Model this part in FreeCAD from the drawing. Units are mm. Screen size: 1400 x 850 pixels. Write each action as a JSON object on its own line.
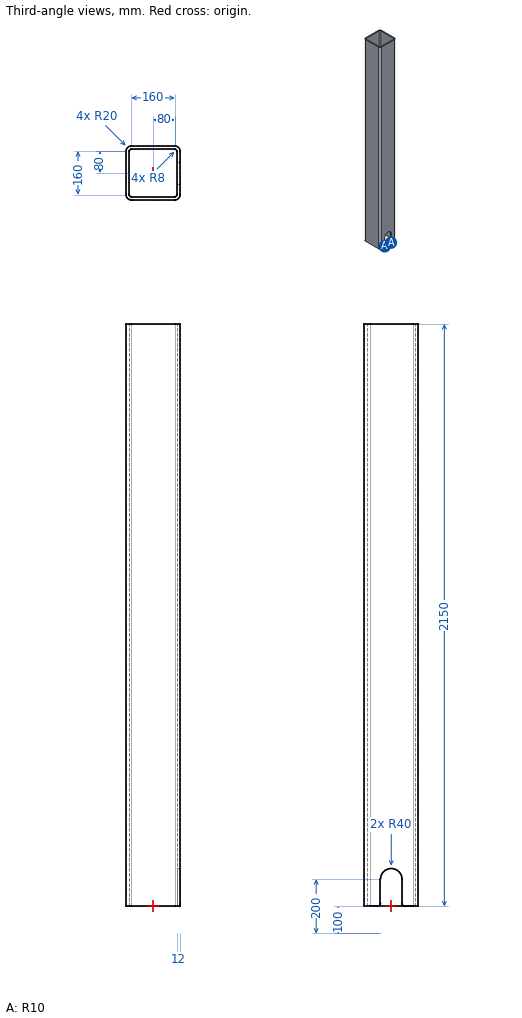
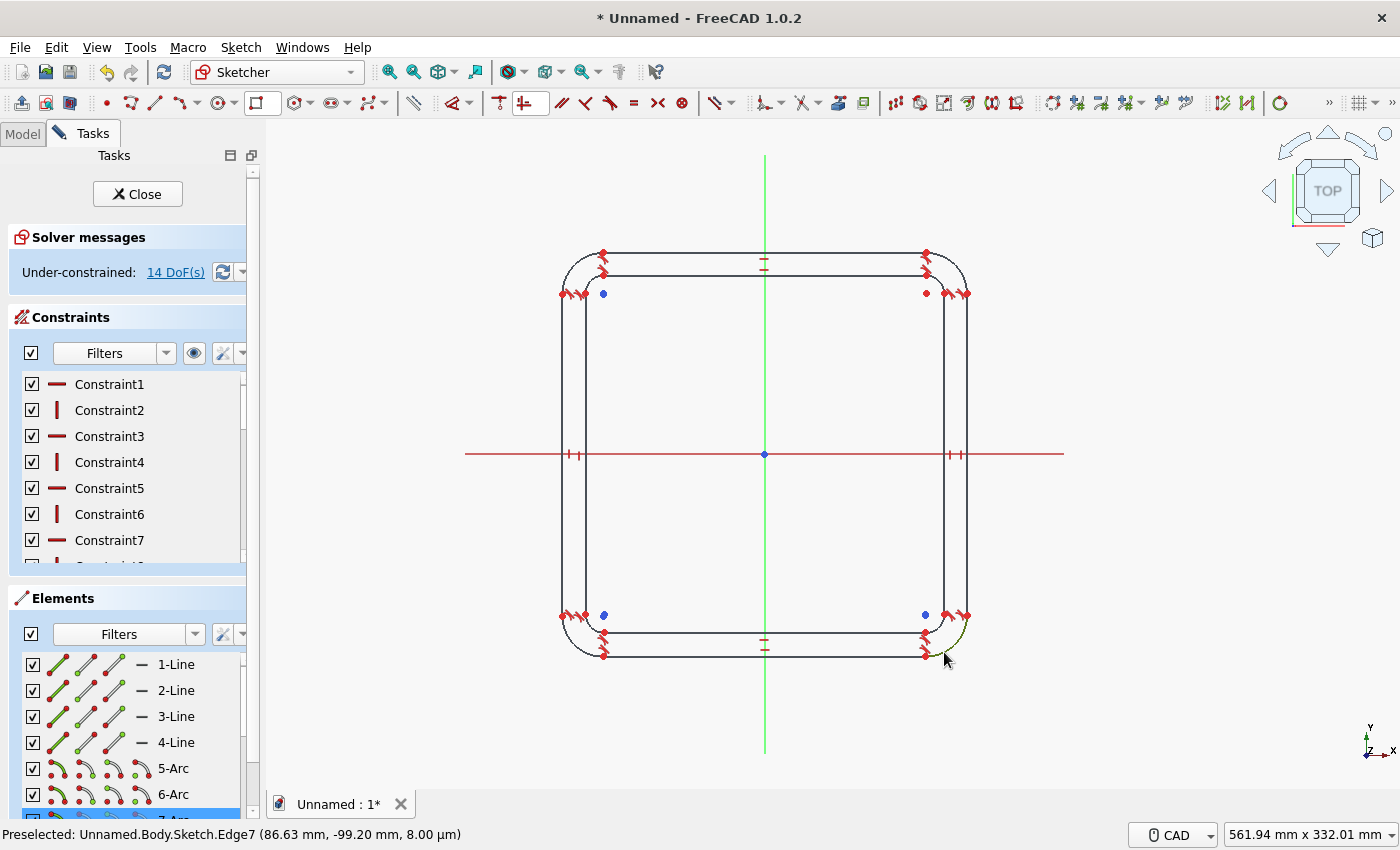
{"action": "left_click", "coordinate": [939, 628]}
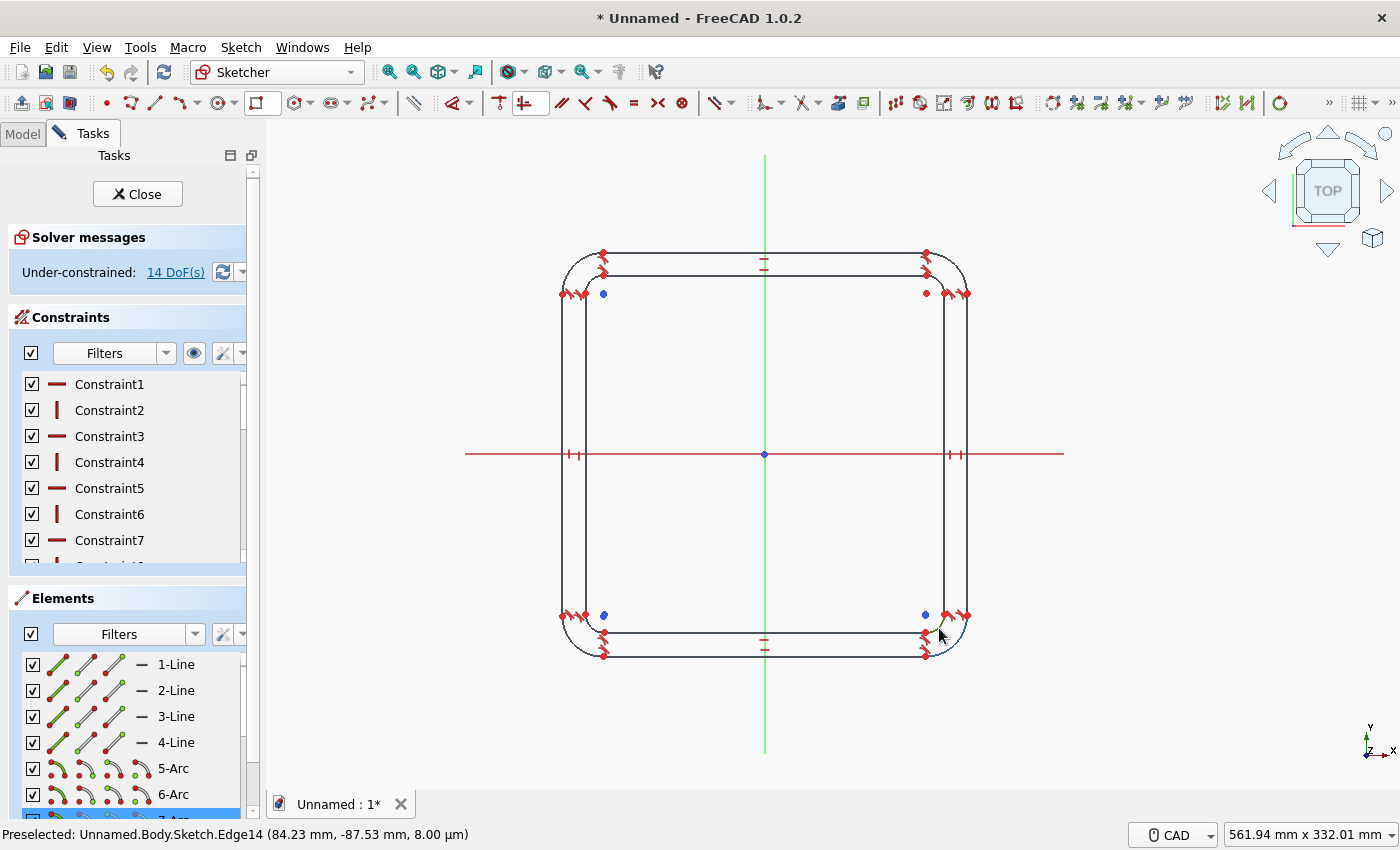
{"action": "left_click", "coordinate": [500, 104]}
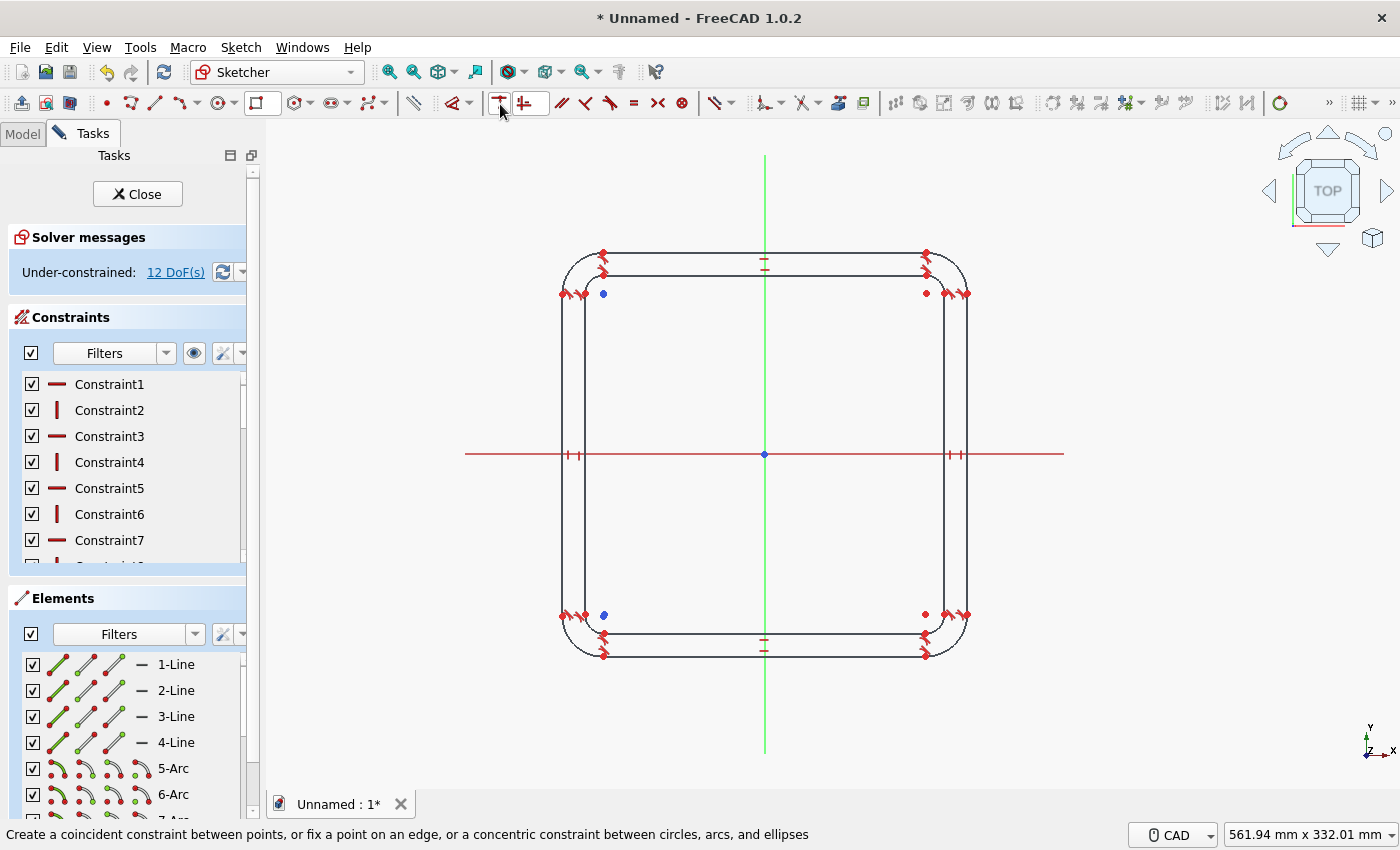
{"action": "left_click", "coordinate": [567, 635]}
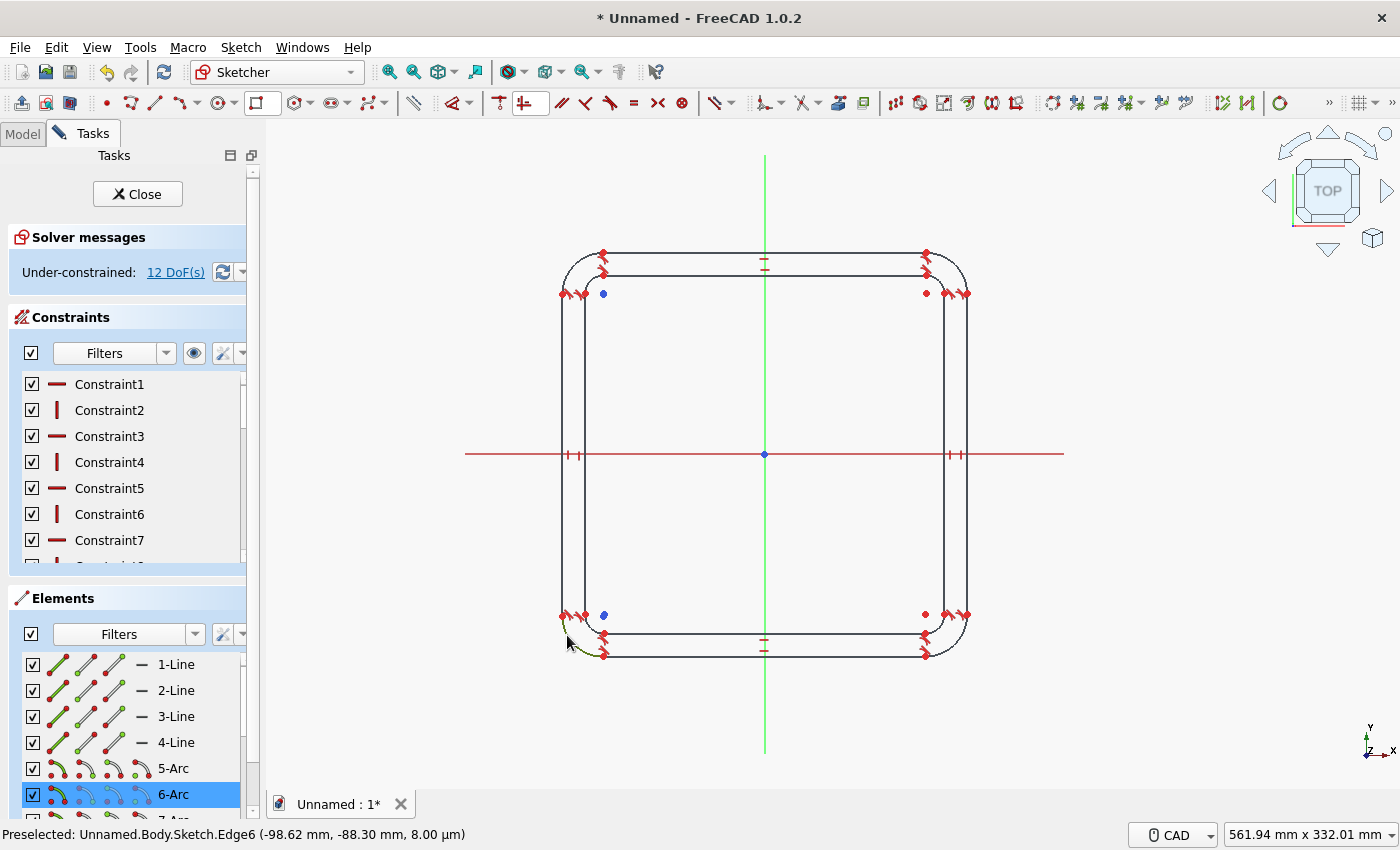
{"action": "scroll", "coordinate": [587, 623], "scroll_direction": "up", "scroll_amount": 3}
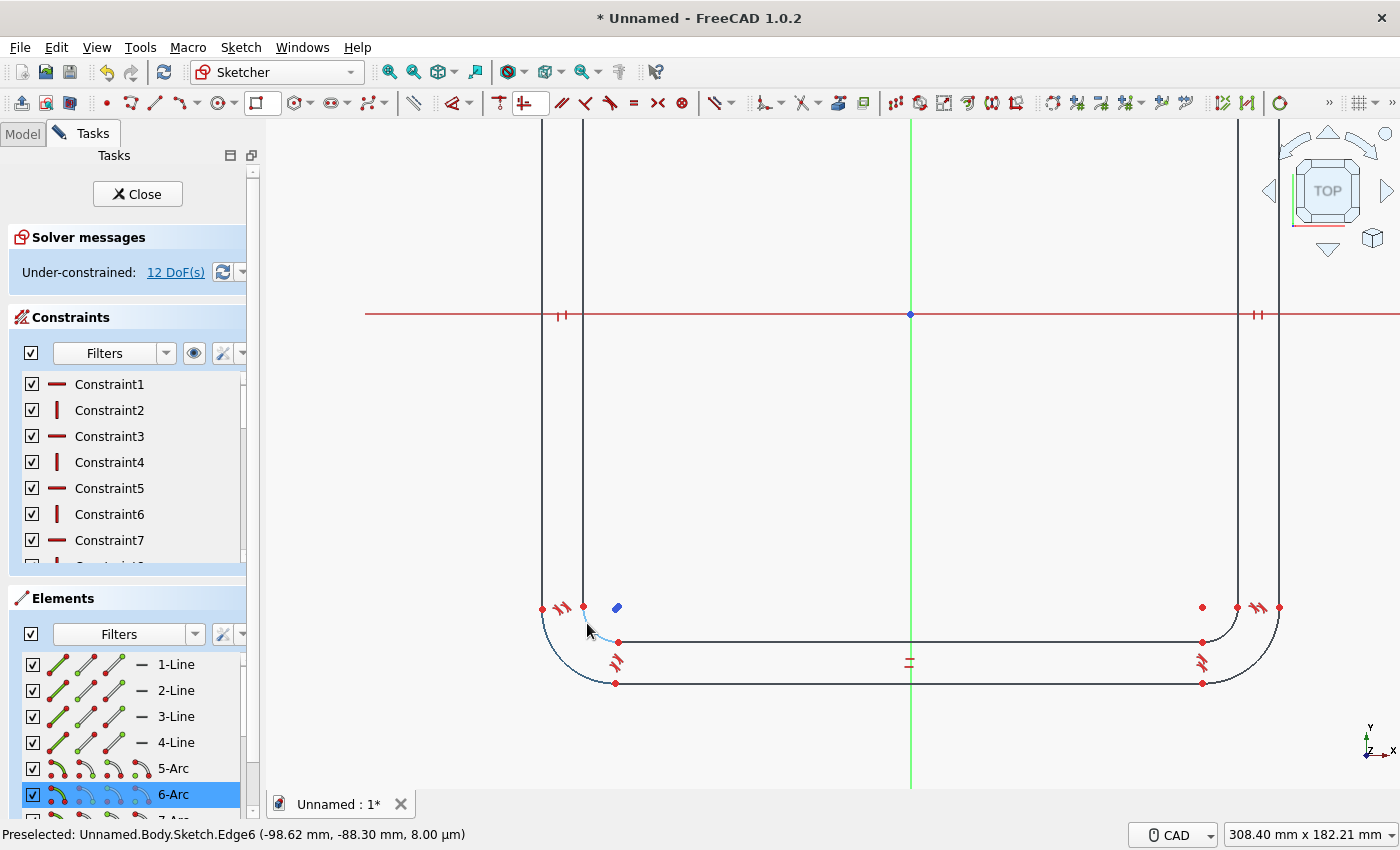
{"action": "left_click", "coordinate": [587, 623]}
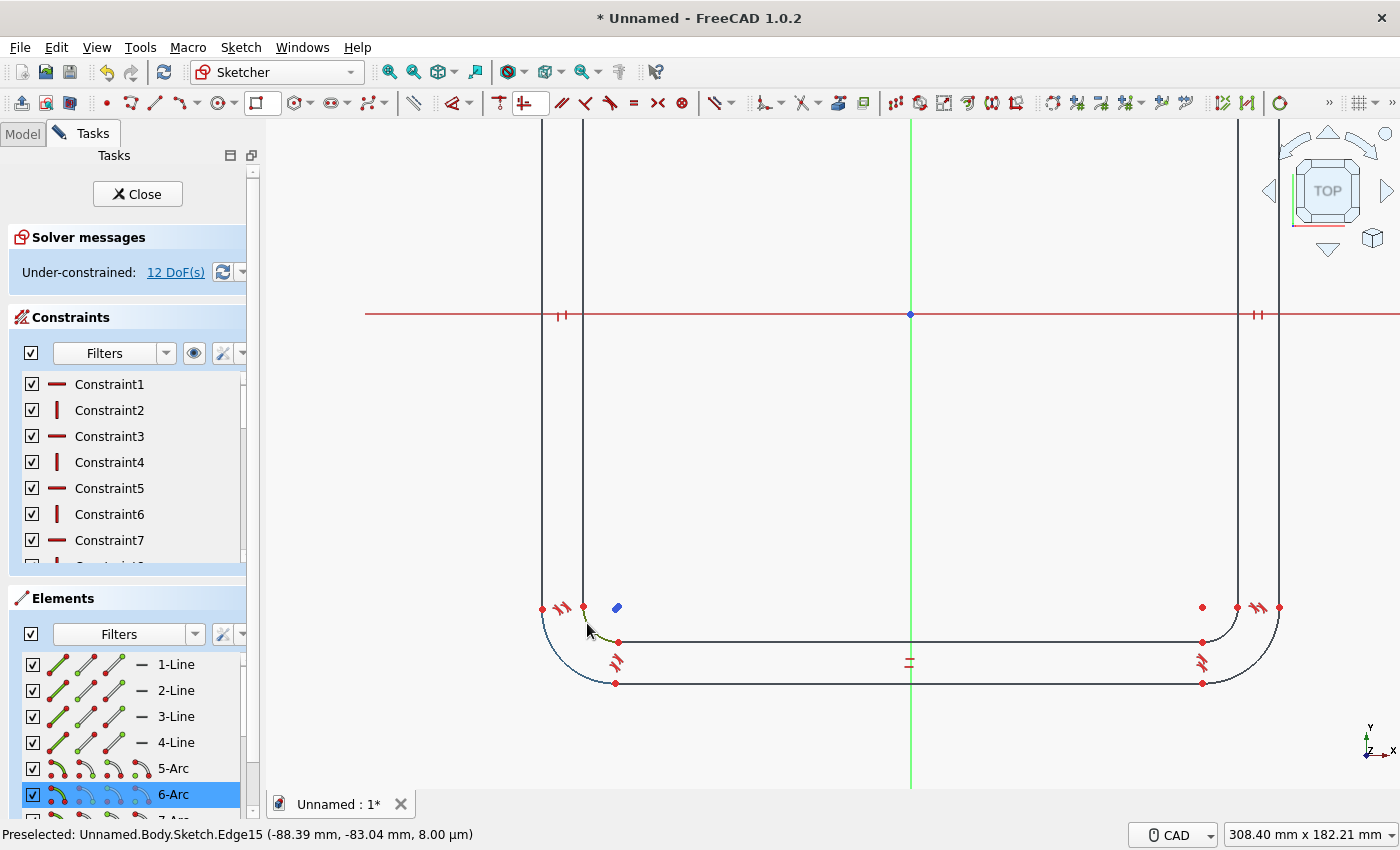
{"action": "left_click", "coordinate": [500, 104]}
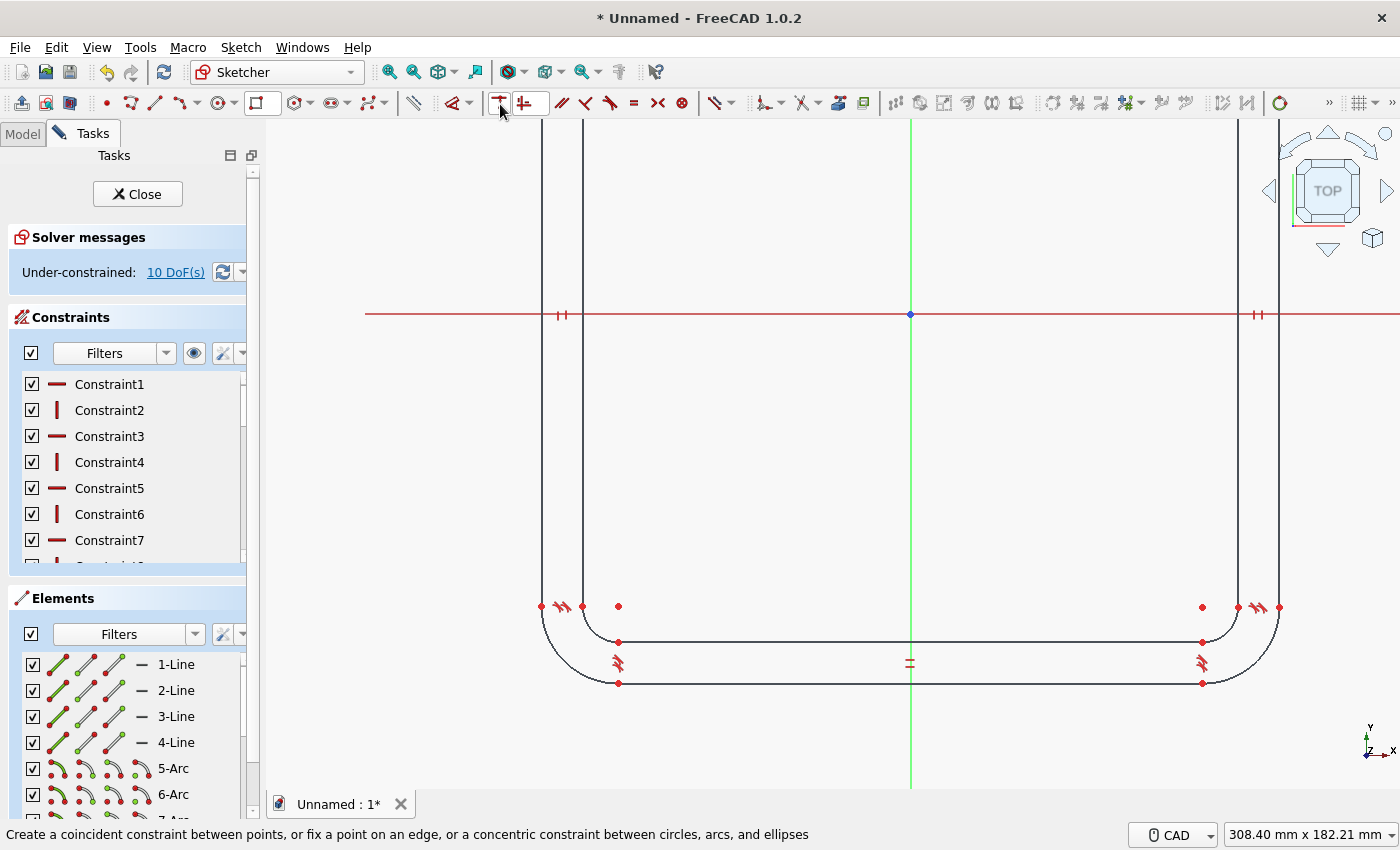
{"action": "scroll", "coordinate": [587, 624], "scroll_direction": "down", "scroll_amount": 3}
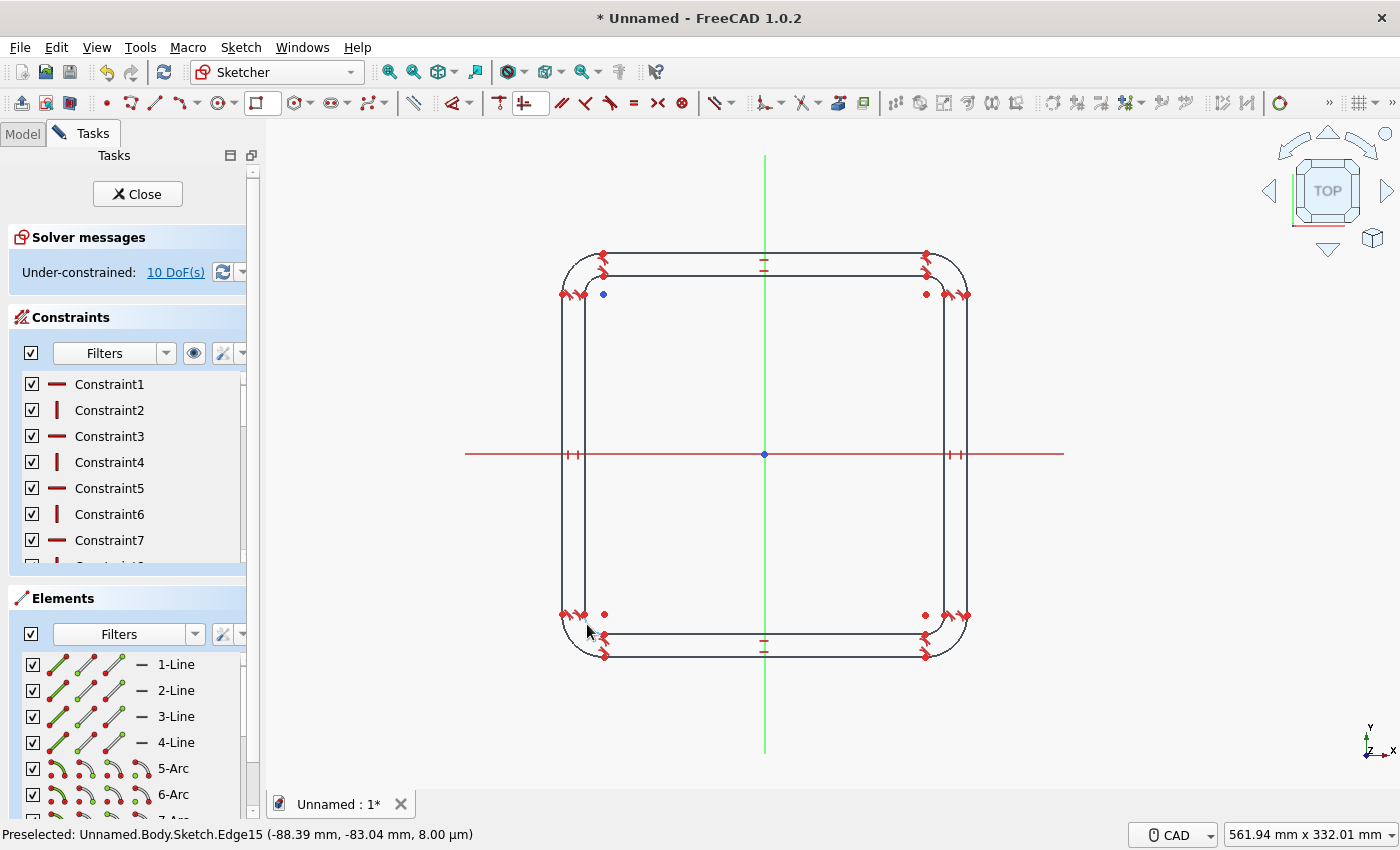
{"action": "left_click", "coordinate": [585, 258]}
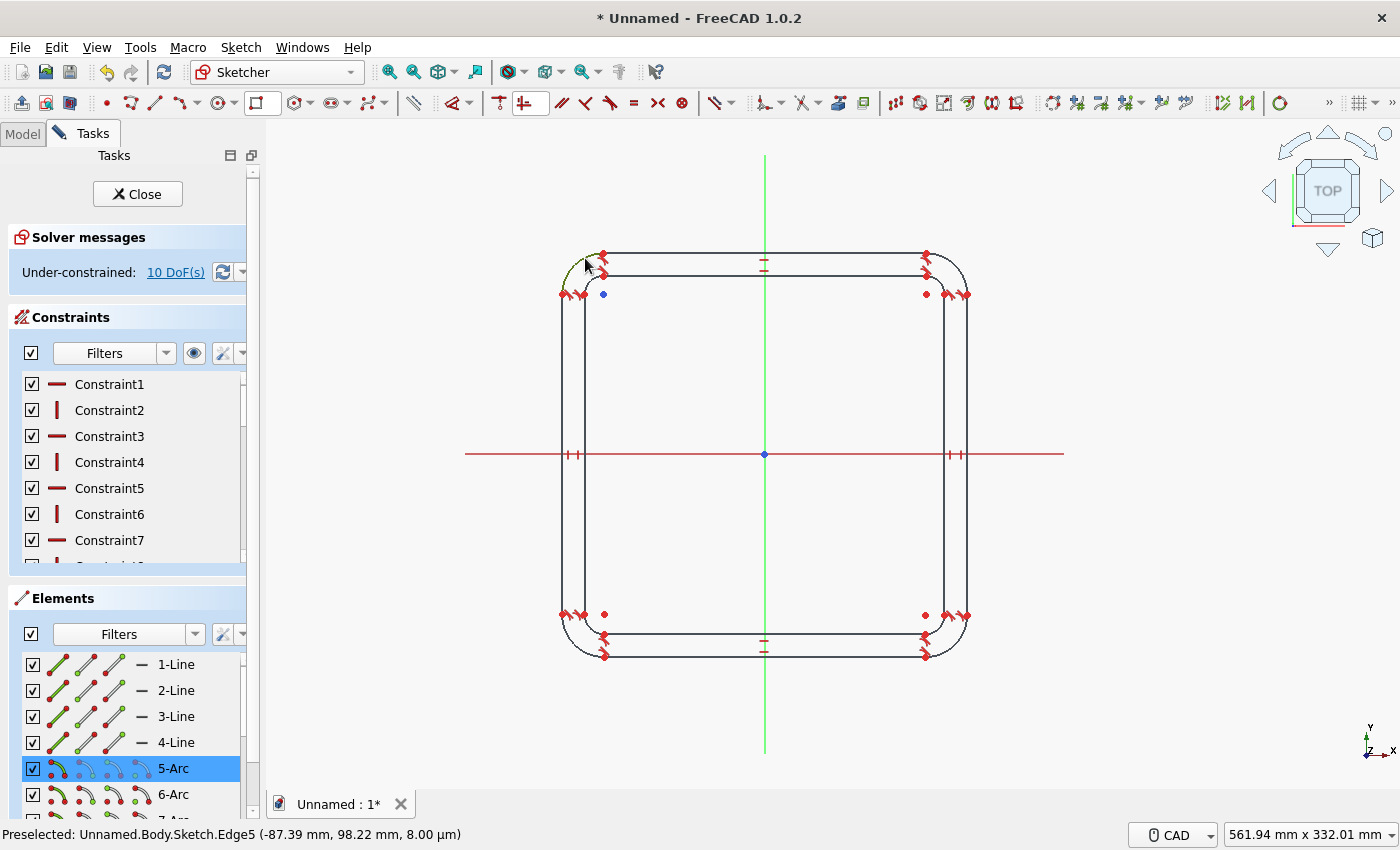
{"action": "left_click", "coordinate": [567, 634]}